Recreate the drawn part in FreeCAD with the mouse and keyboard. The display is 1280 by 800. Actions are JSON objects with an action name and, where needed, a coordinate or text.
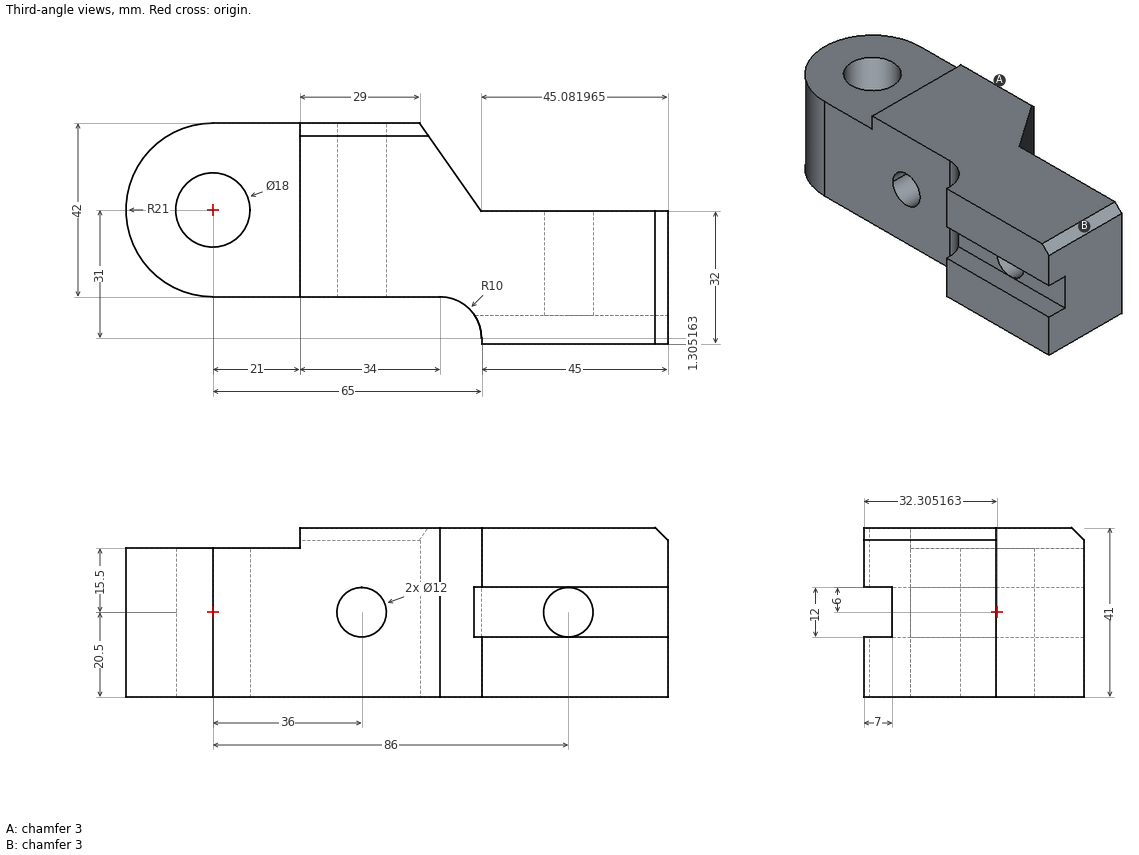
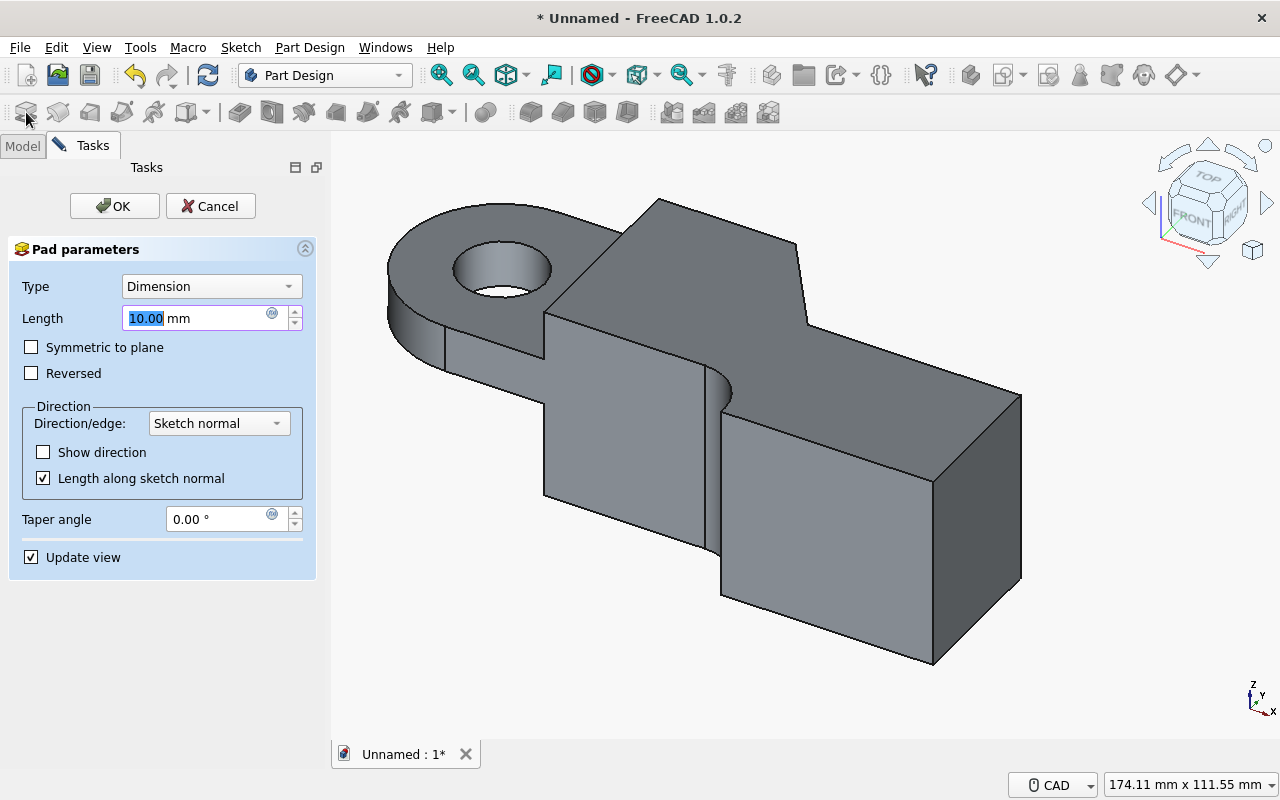
{"action": "left_click", "coordinate": [212, 286]}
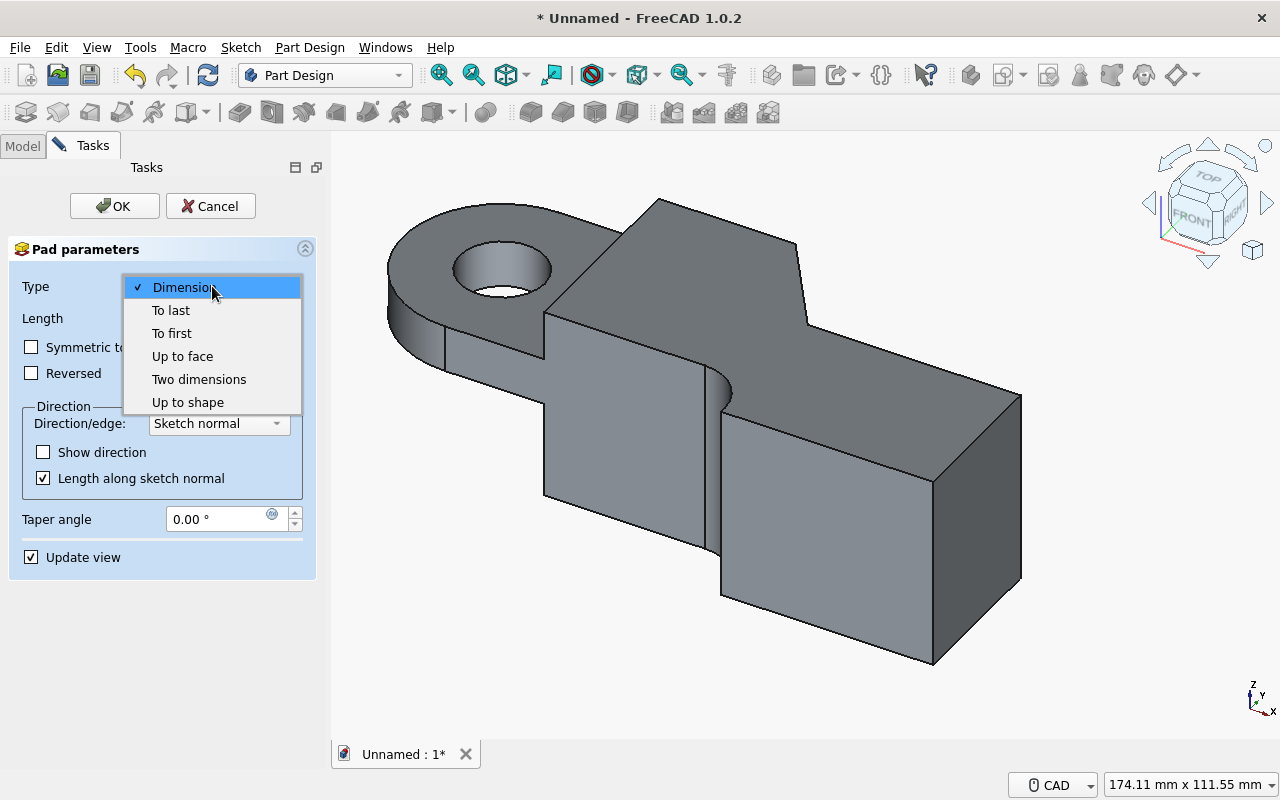
{"action": "left_click", "coordinate": [212, 380]}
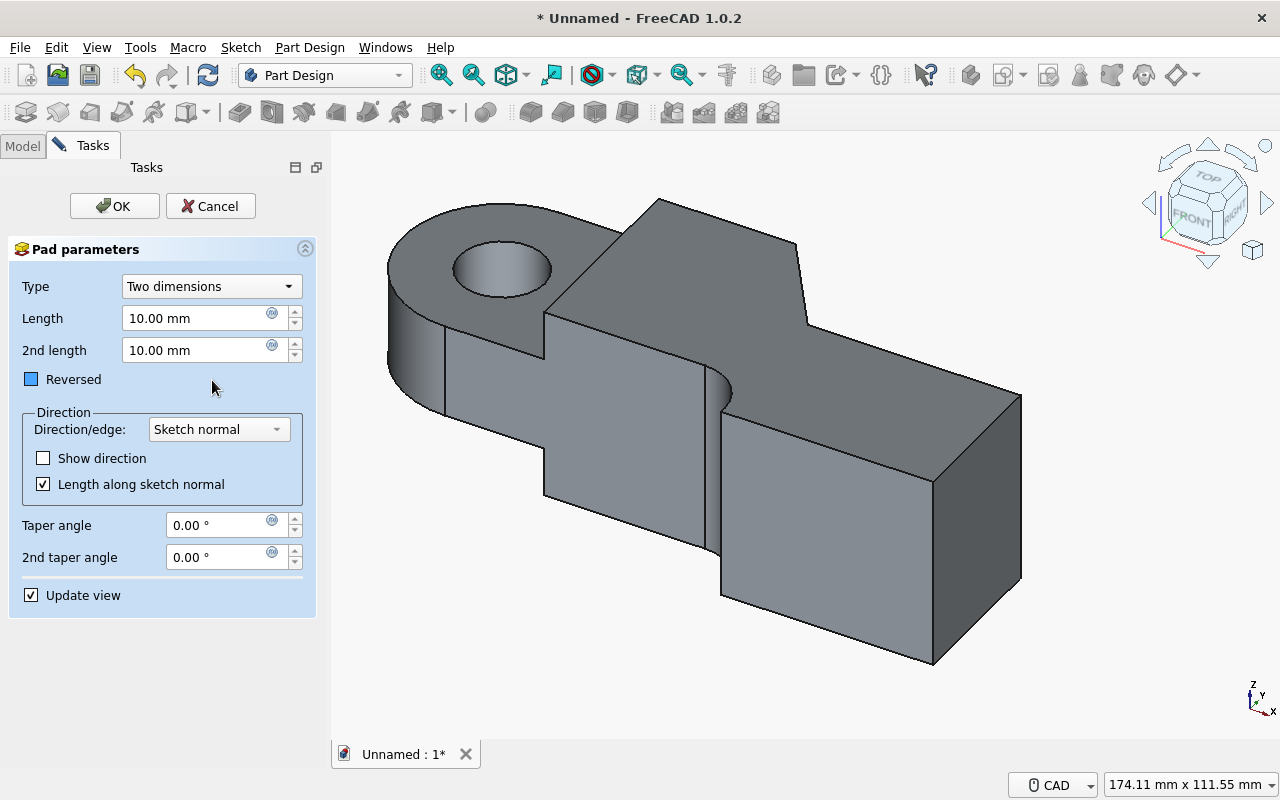
{"action": "triple_click", "coordinate": [204, 318]}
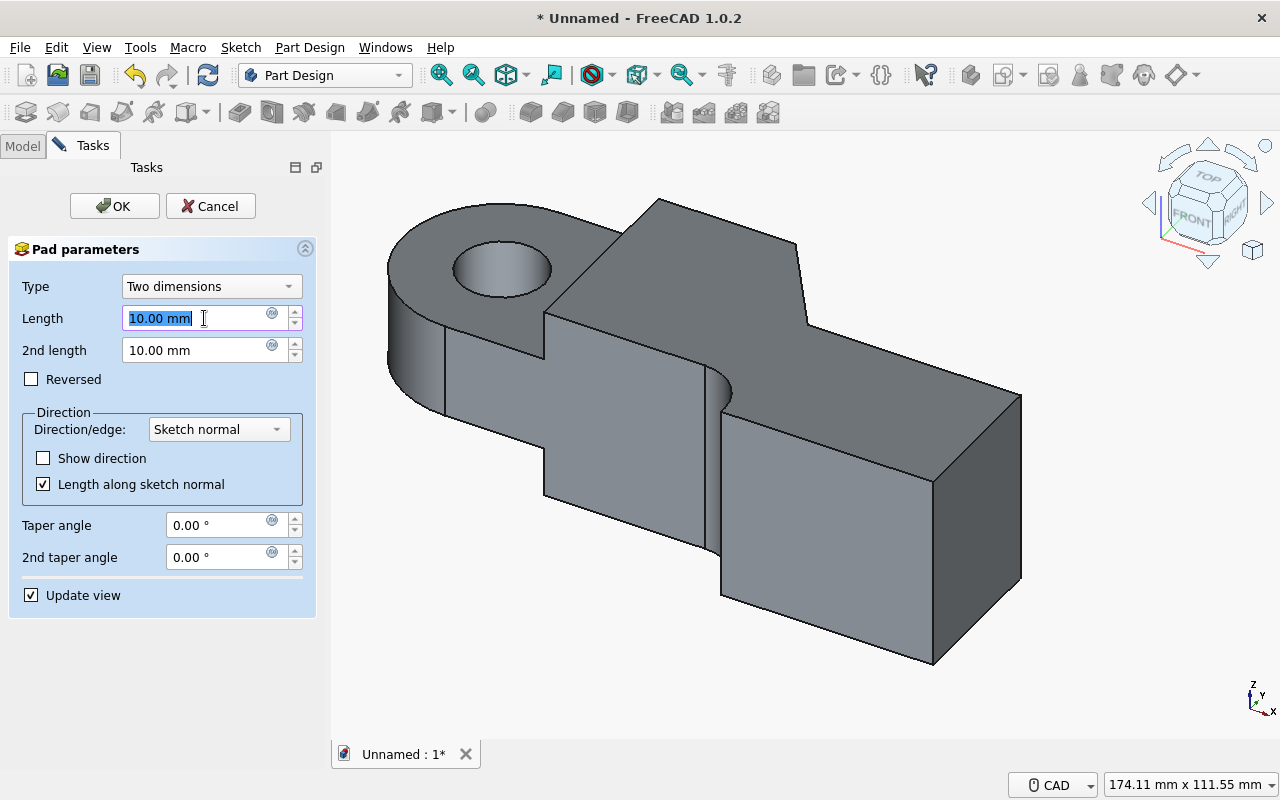
{"action": "type", "text": "15.5"}
{"action": "key", "text": "Tab"}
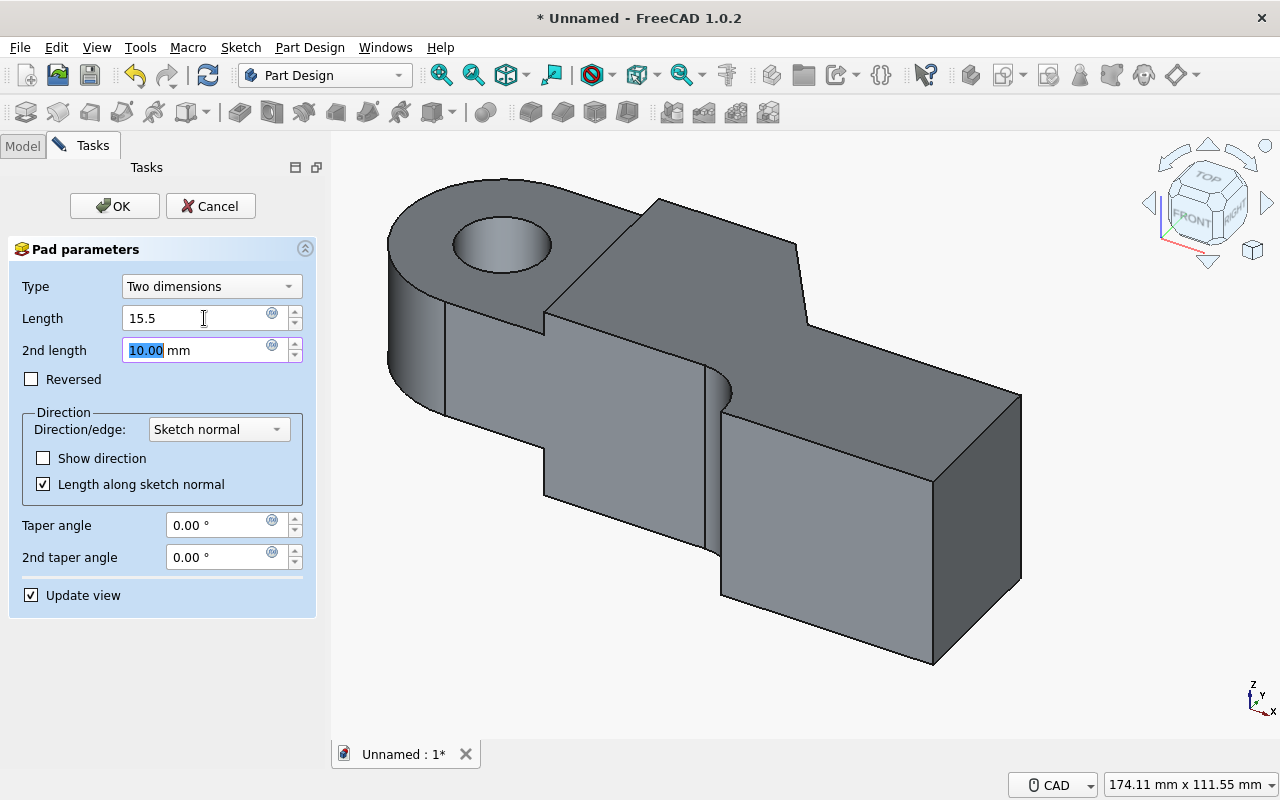
{"action": "type", "text": "20.5"}
{"action": "key", "text": "Tab"}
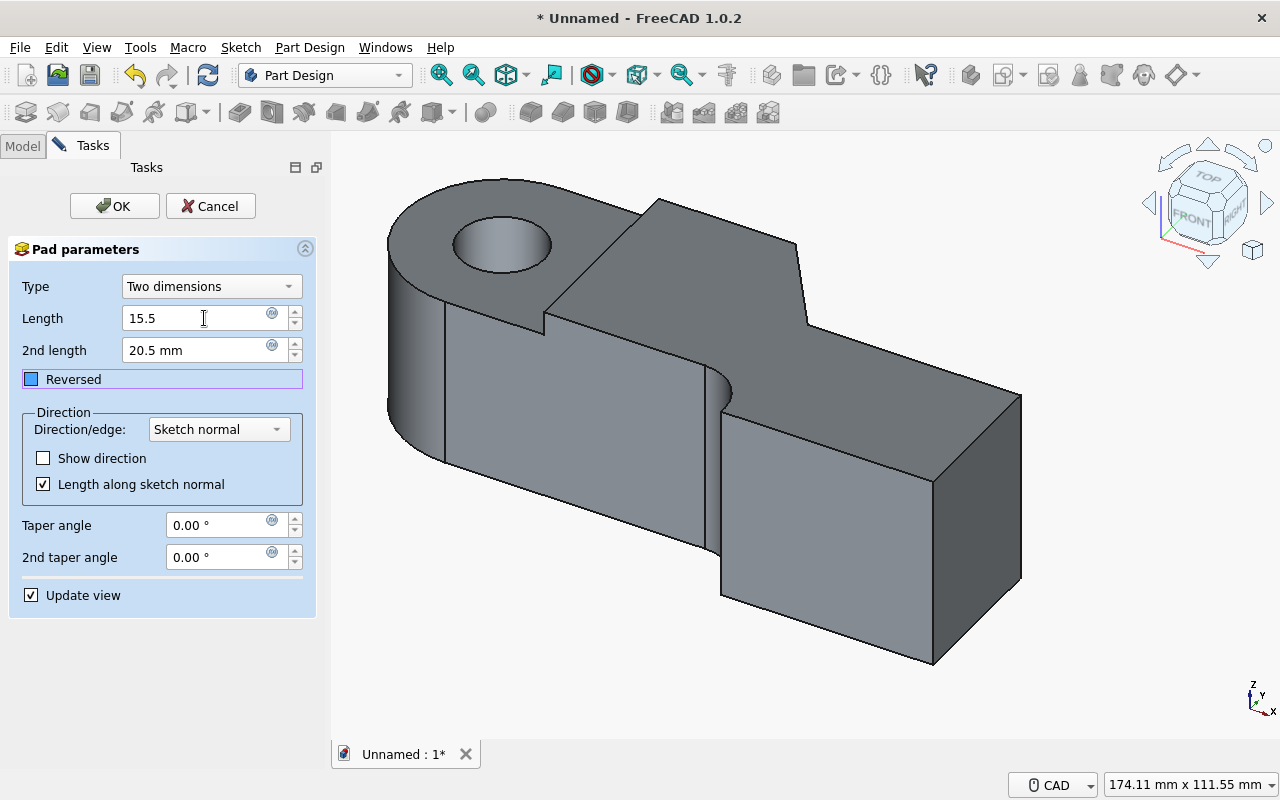
{"action": "left_click", "coordinate": [115, 206]}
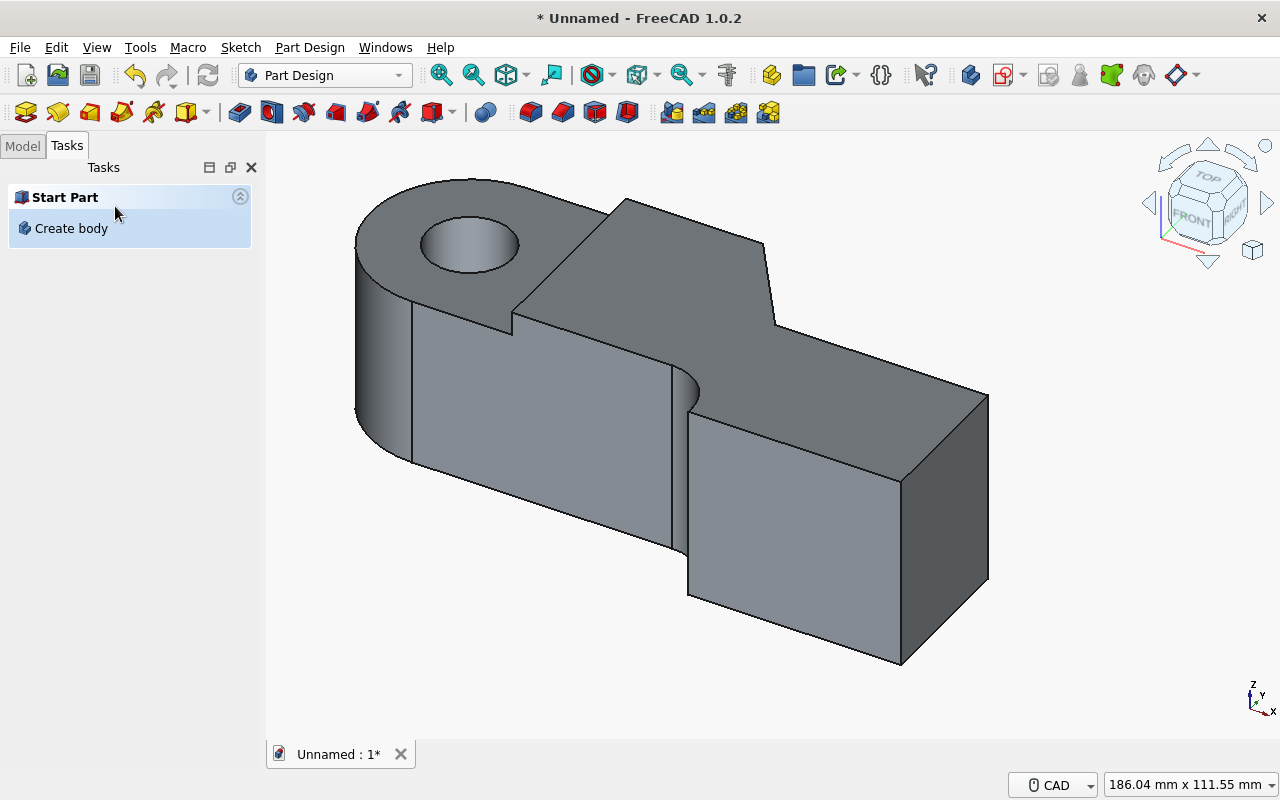
{"action": "key", "text": "0"}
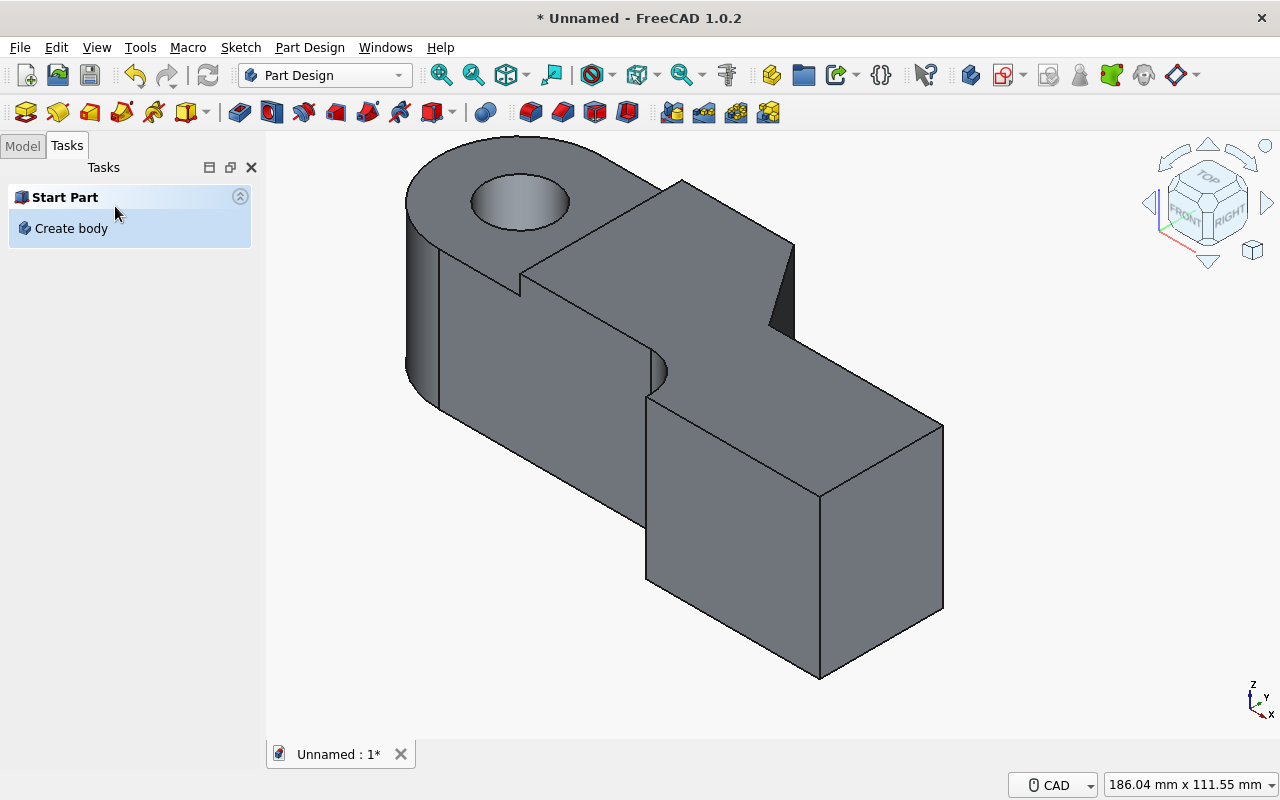
{"action": "left_click", "coordinate": [442, 76]}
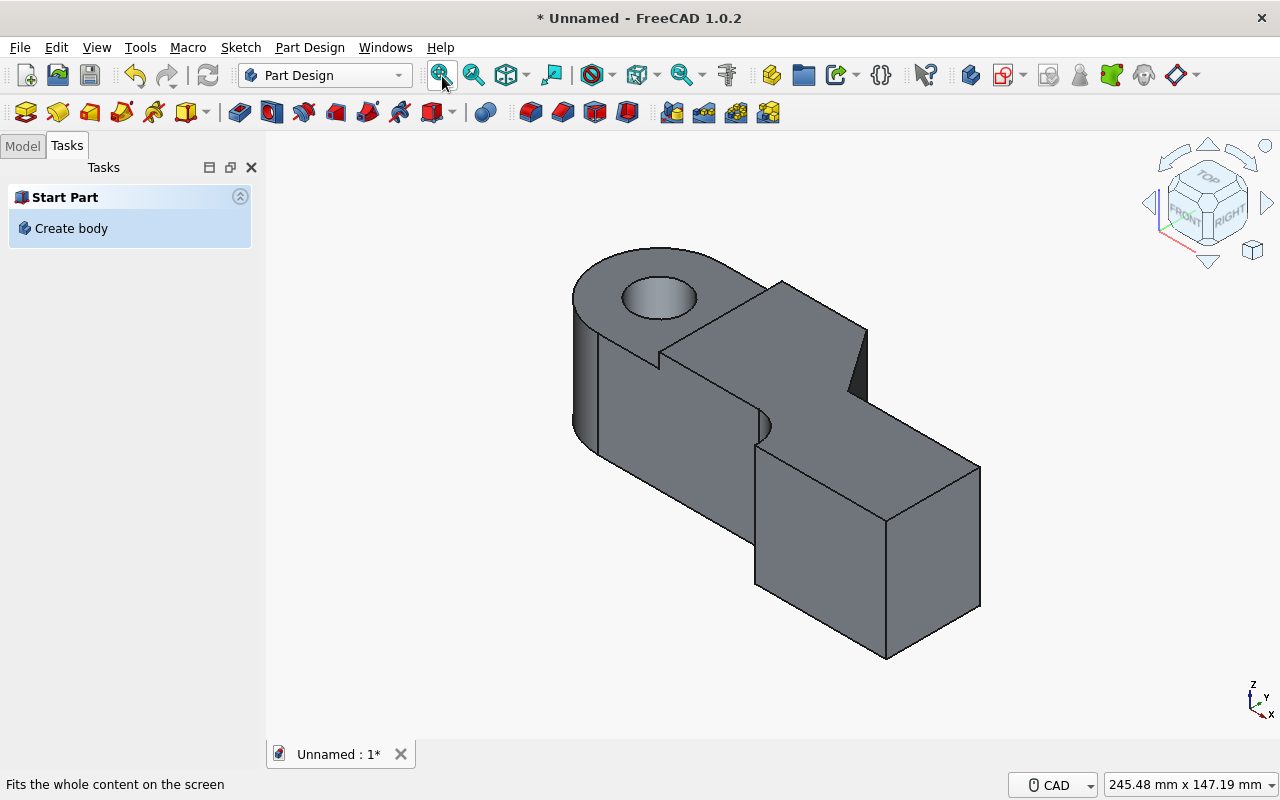
{"action": "key", "text": "2"}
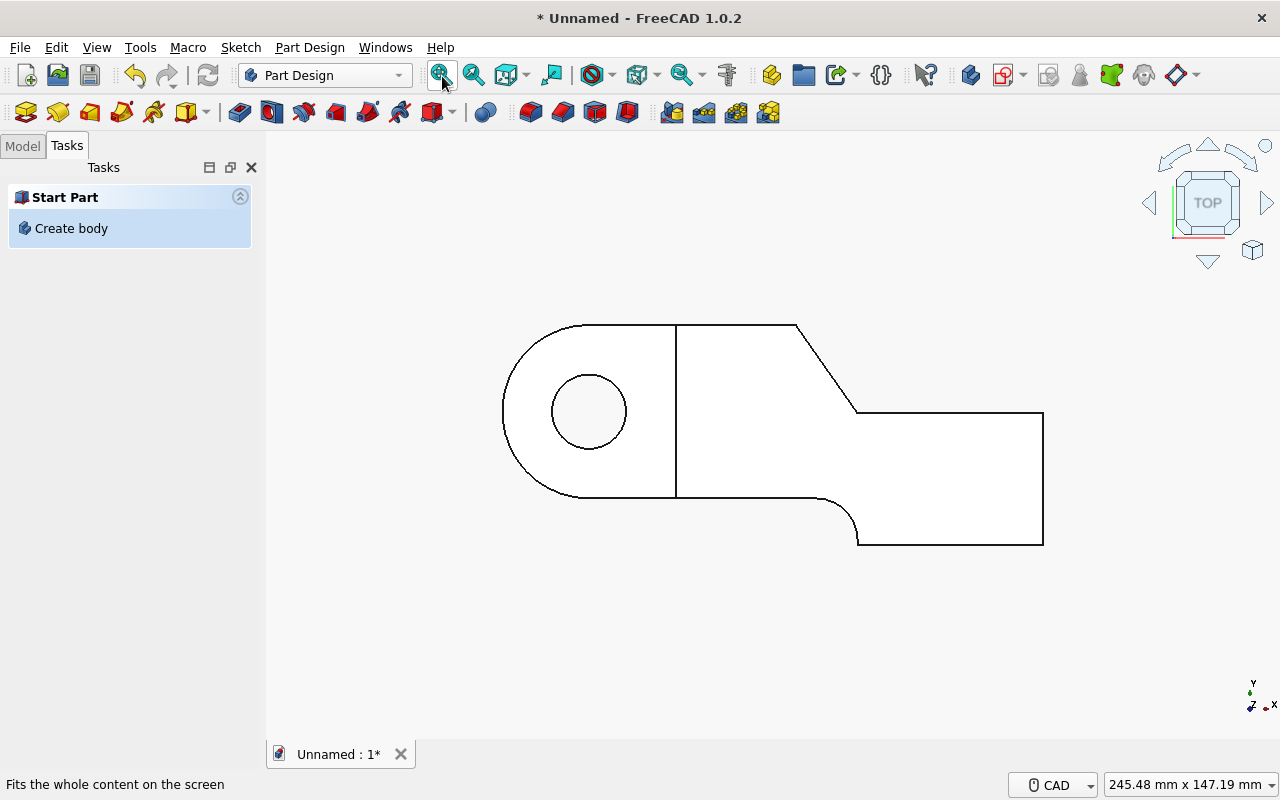
{"action": "left_click", "coordinate": [736, 324]}